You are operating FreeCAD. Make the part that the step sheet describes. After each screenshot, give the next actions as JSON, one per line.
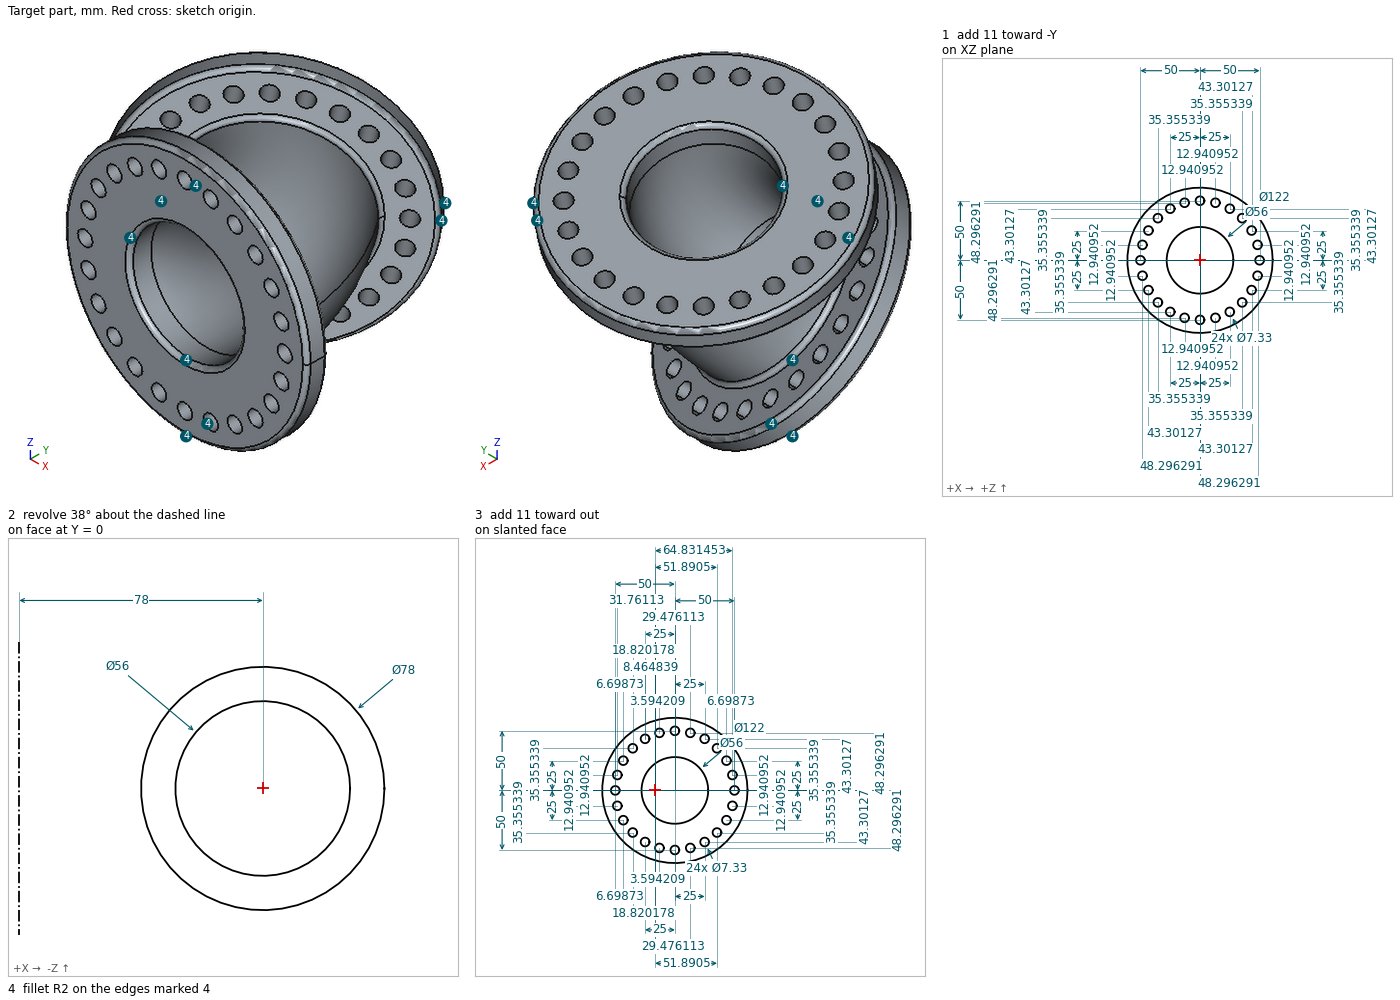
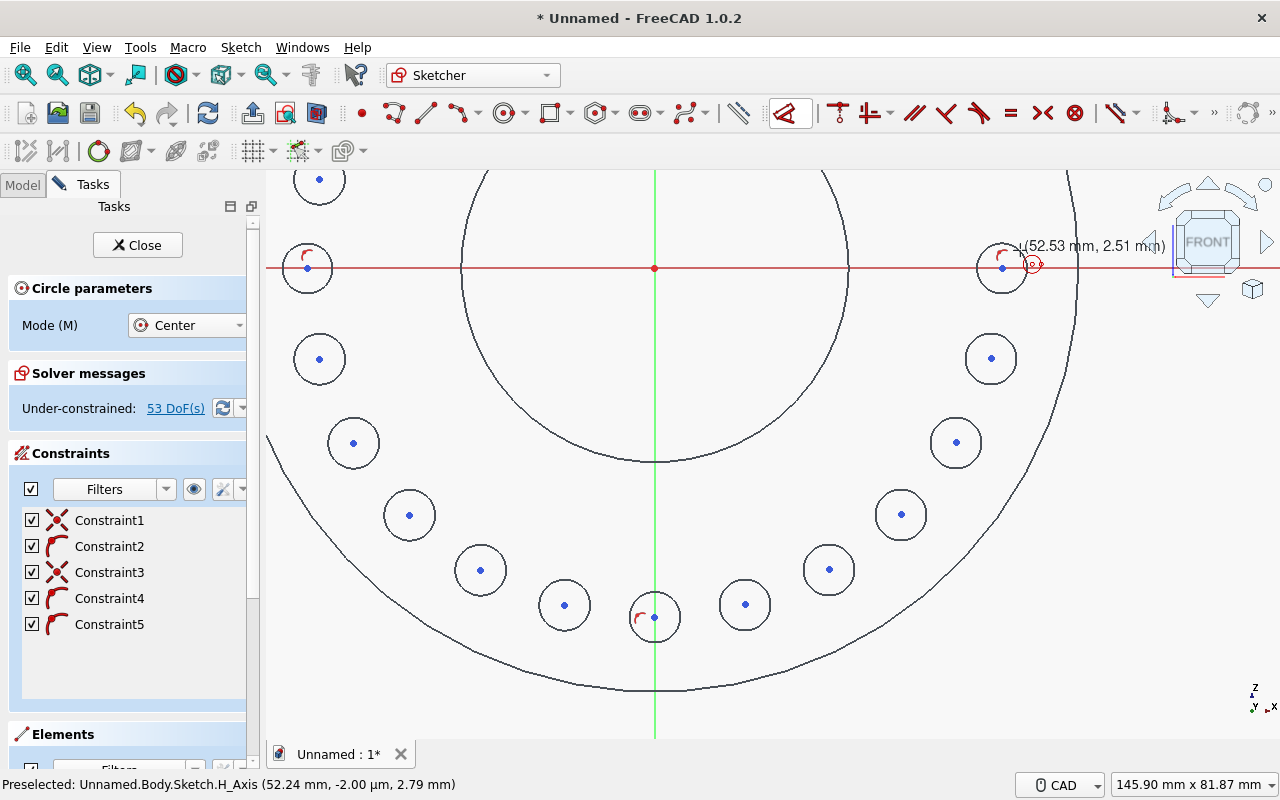
{"action": "scroll", "coordinate": [745, 606], "scroll_direction": "down", "scroll_amount": 4}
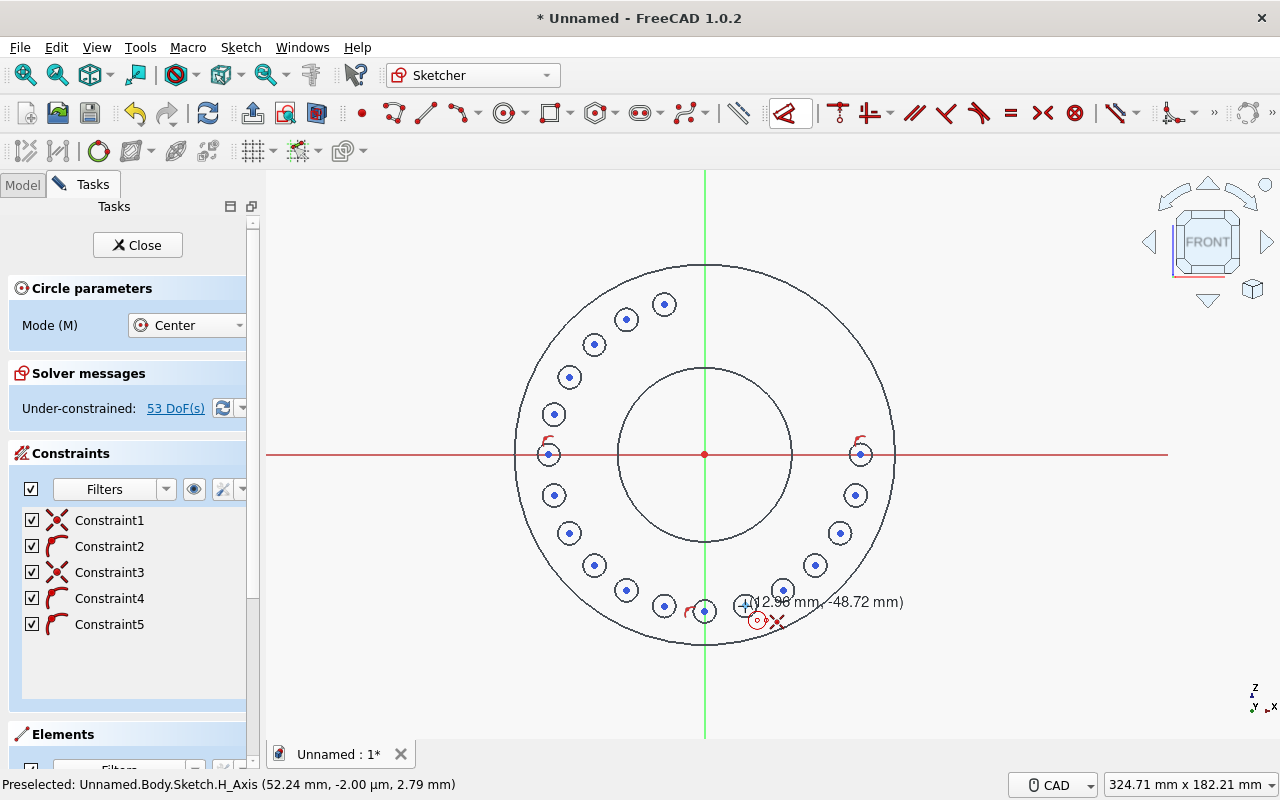
{"action": "scroll", "coordinate": [705, 299], "scroll_direction": "up", "scroll_amount": 4}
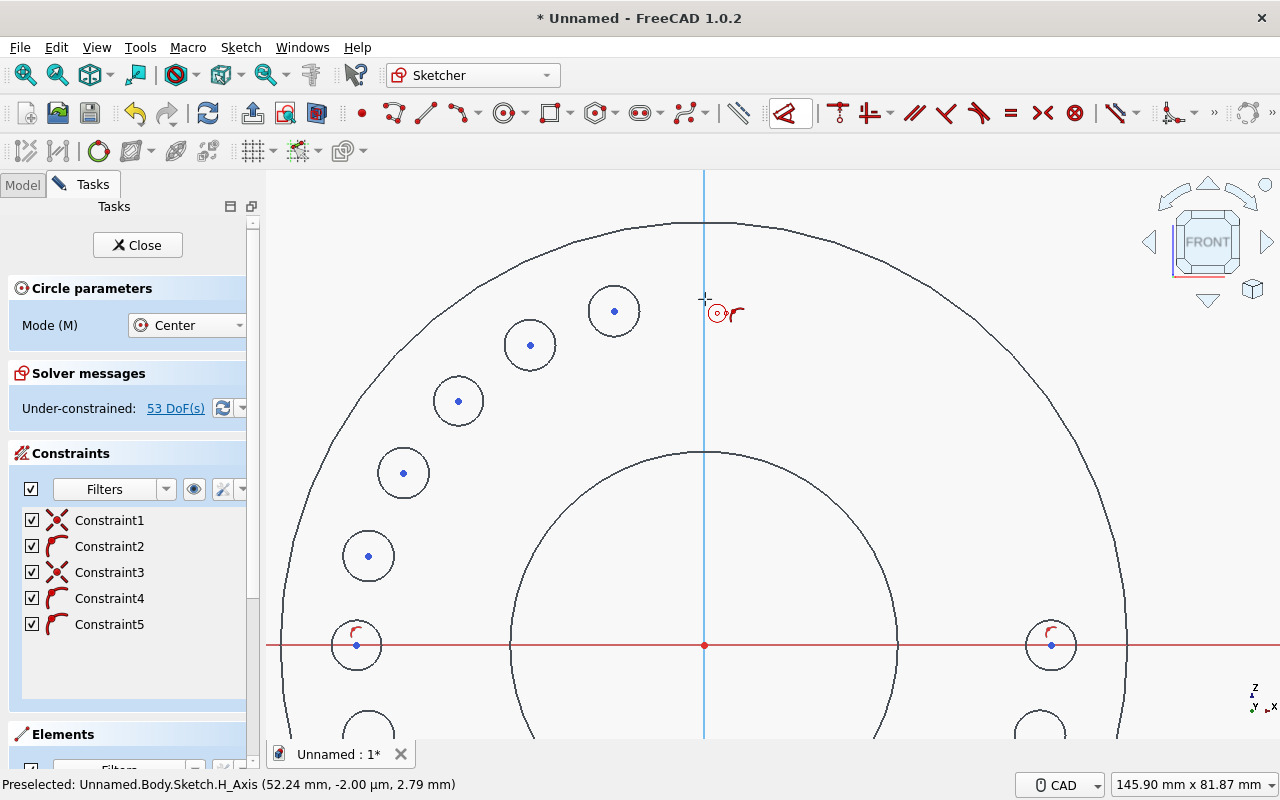
{"action": "left_click", "coordinate": [704, 298]}
{"action": "left_click", "coordinate": [722, 280]}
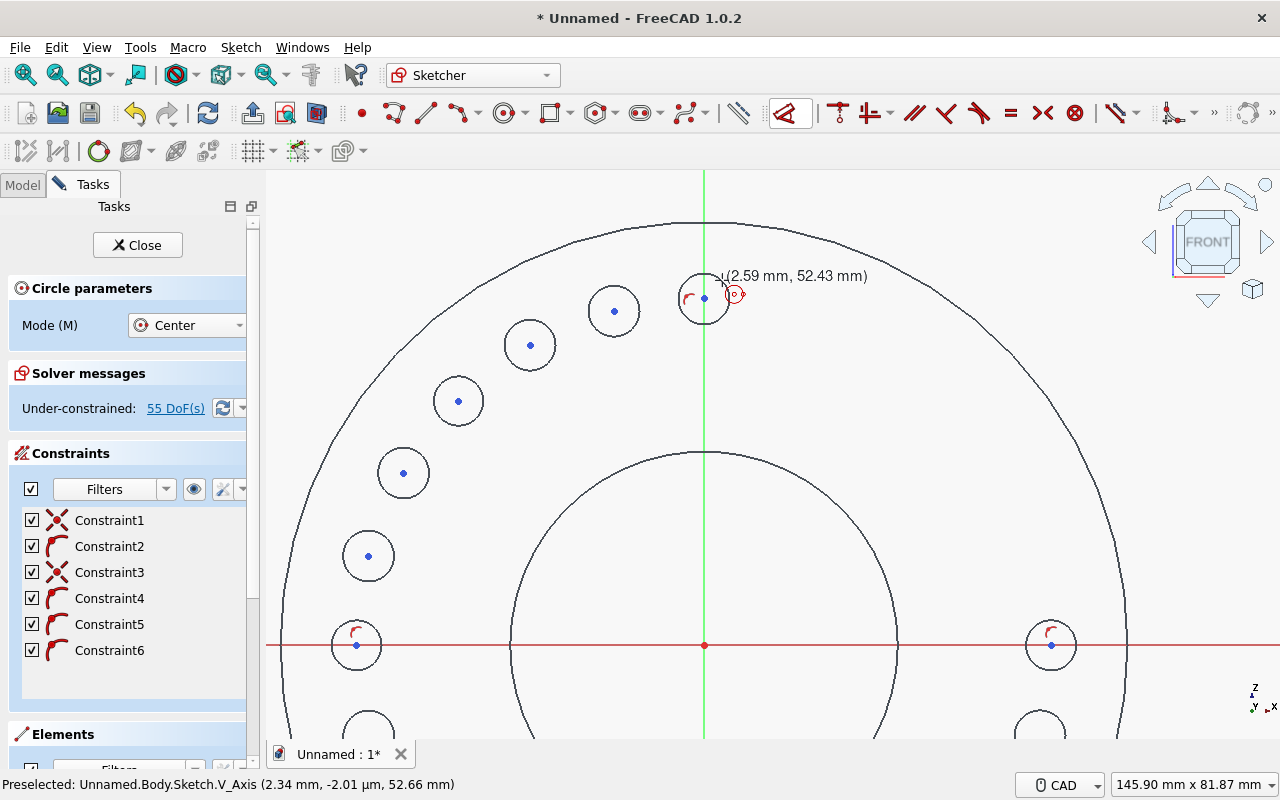
{"action": "left_click", "coordinate": [794, 310]}
{"action": "left_click", "coordinate": [812, 292]}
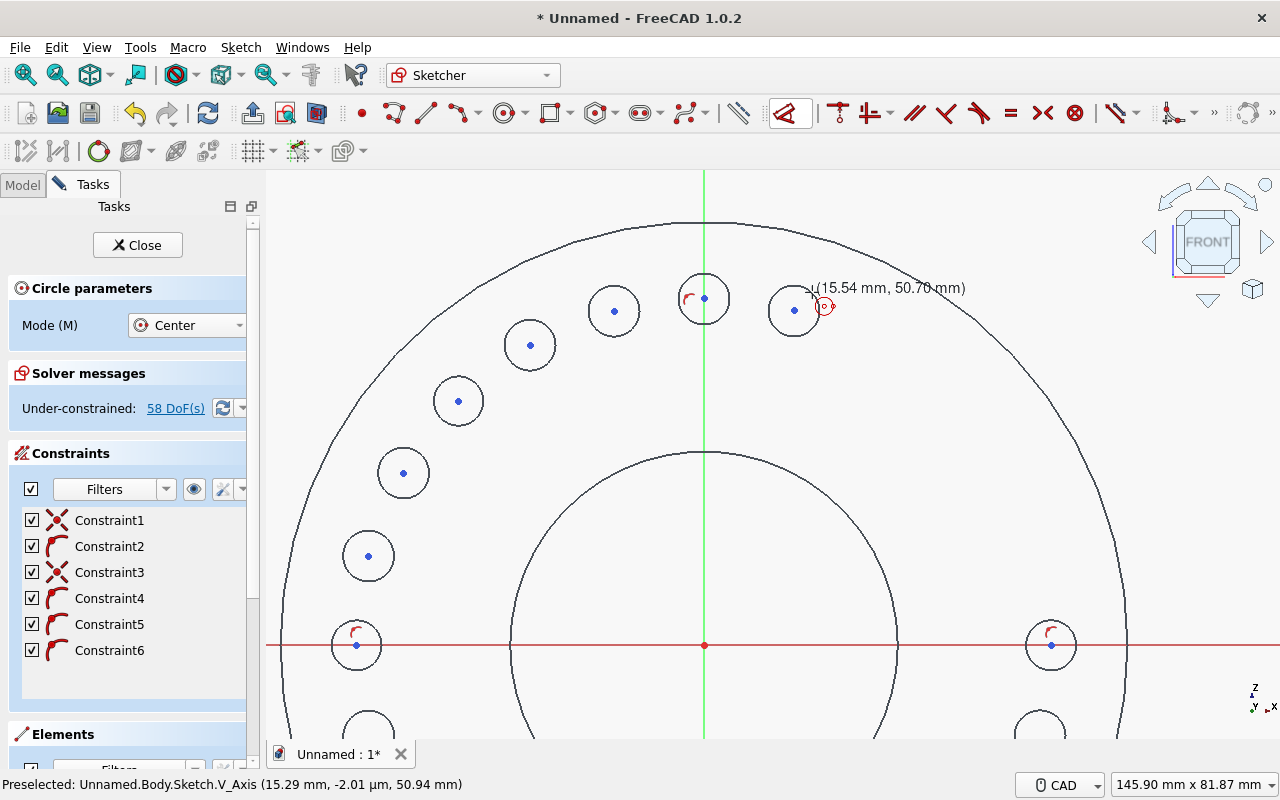
{"action": "left_click", "coordinate": [878, 344]}
{"action": "left_click", "coordinate": [896, 326]}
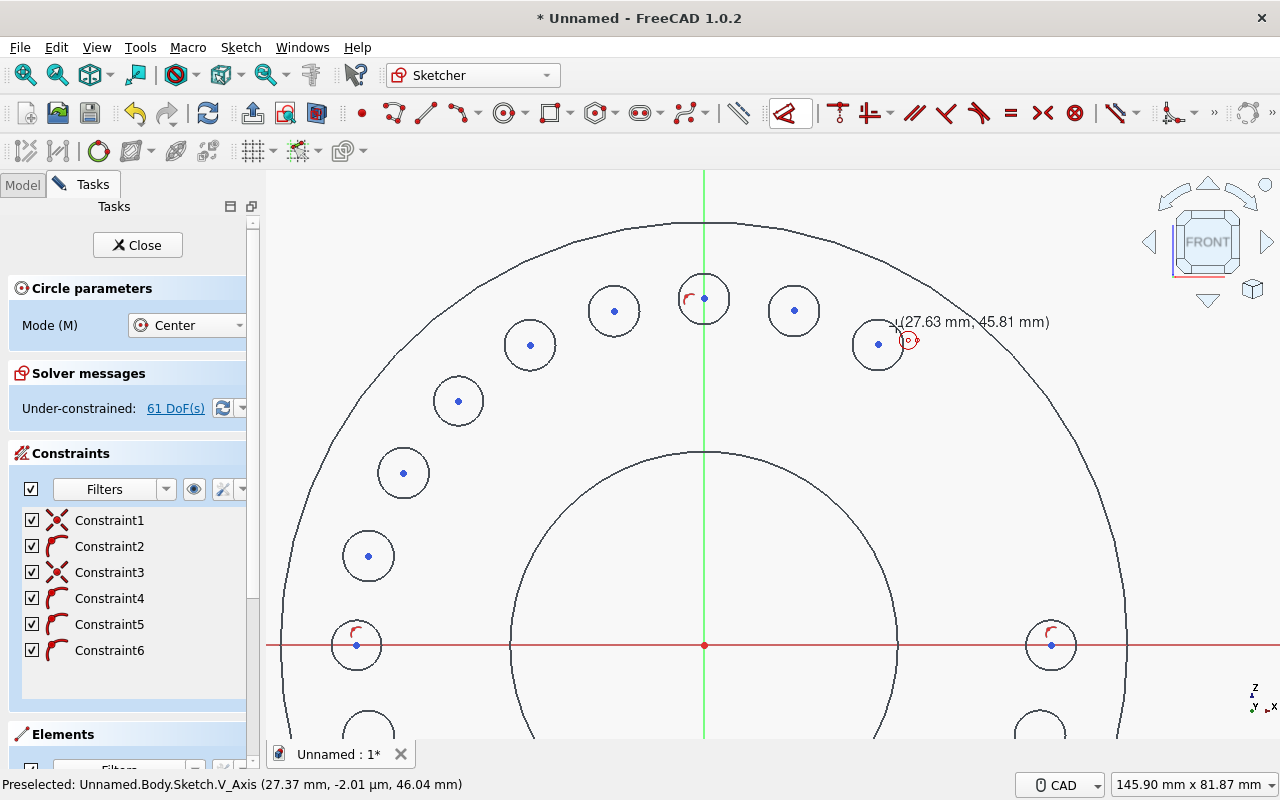
{"action": "left_click", "coordinate": [1040, 555]}
{"action": "left_click", "coordinate": [1058, 537]}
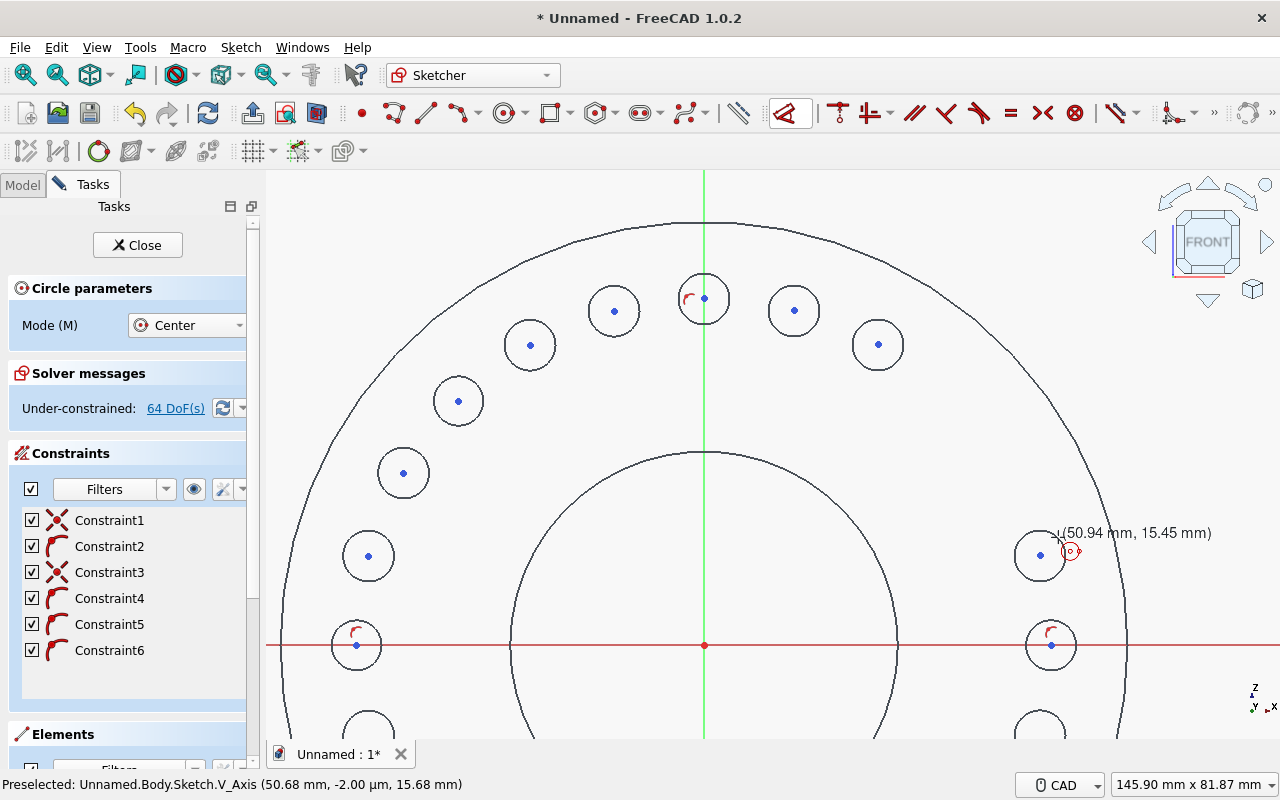
{"action": "left_click", "coordinate": [1005, 472]}
{"action": "left_click", "coordinate": [1023, 454]}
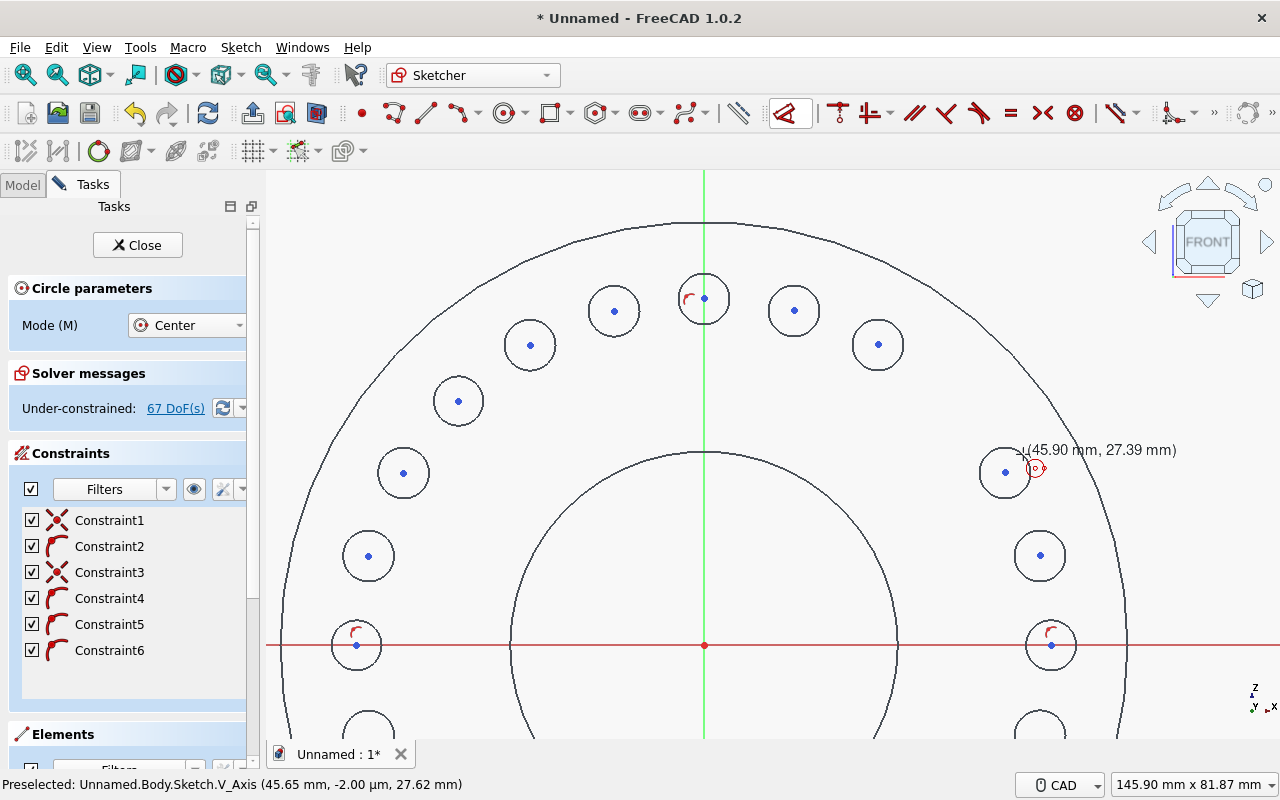
{"action": "left_click", "coordinate": [950, 400]}
{"action": "left_click", "coordinate": [968, 382]}
{"action": "key", "text": "Escape"}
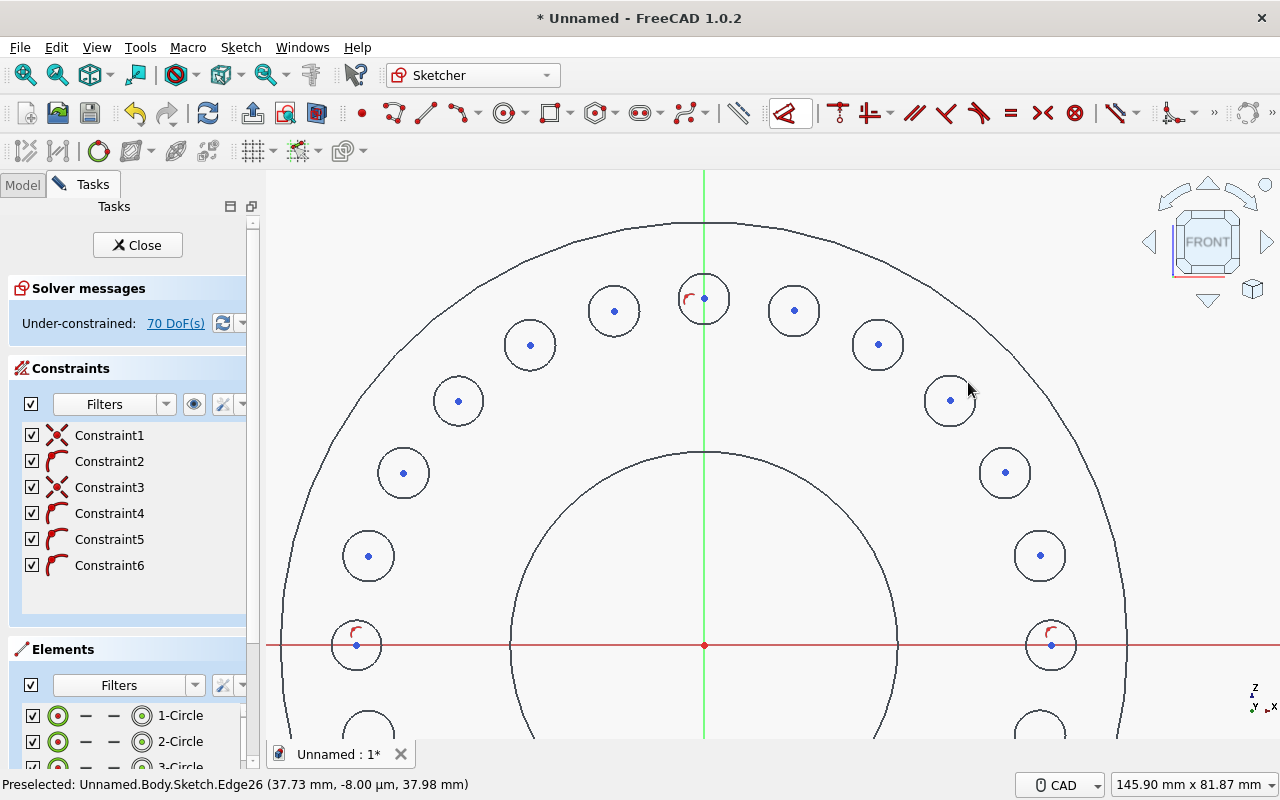
{"action": "scroll", "coordinate": [705, 299], "scroll_direction": "down", "scroll_amount": 4}